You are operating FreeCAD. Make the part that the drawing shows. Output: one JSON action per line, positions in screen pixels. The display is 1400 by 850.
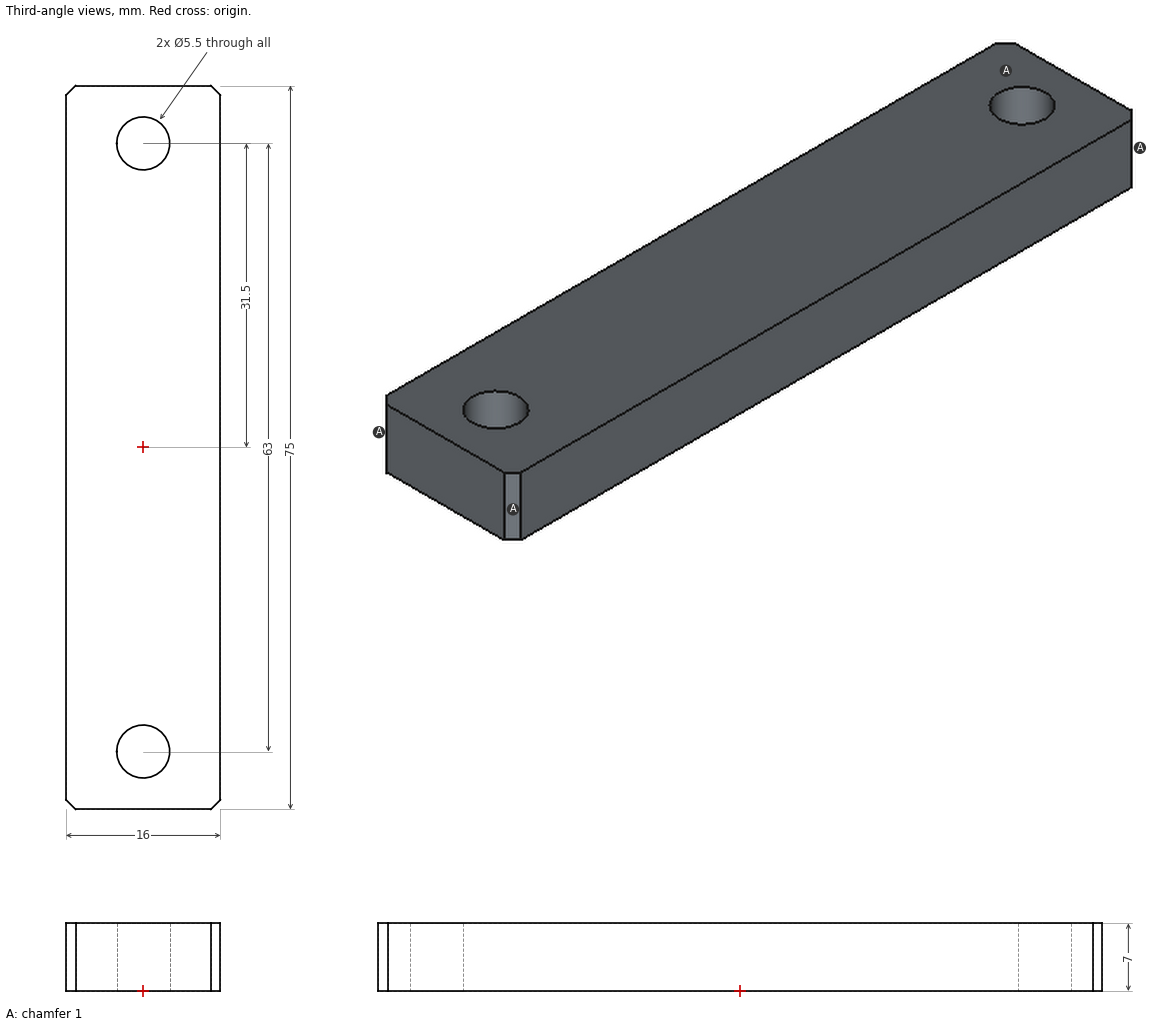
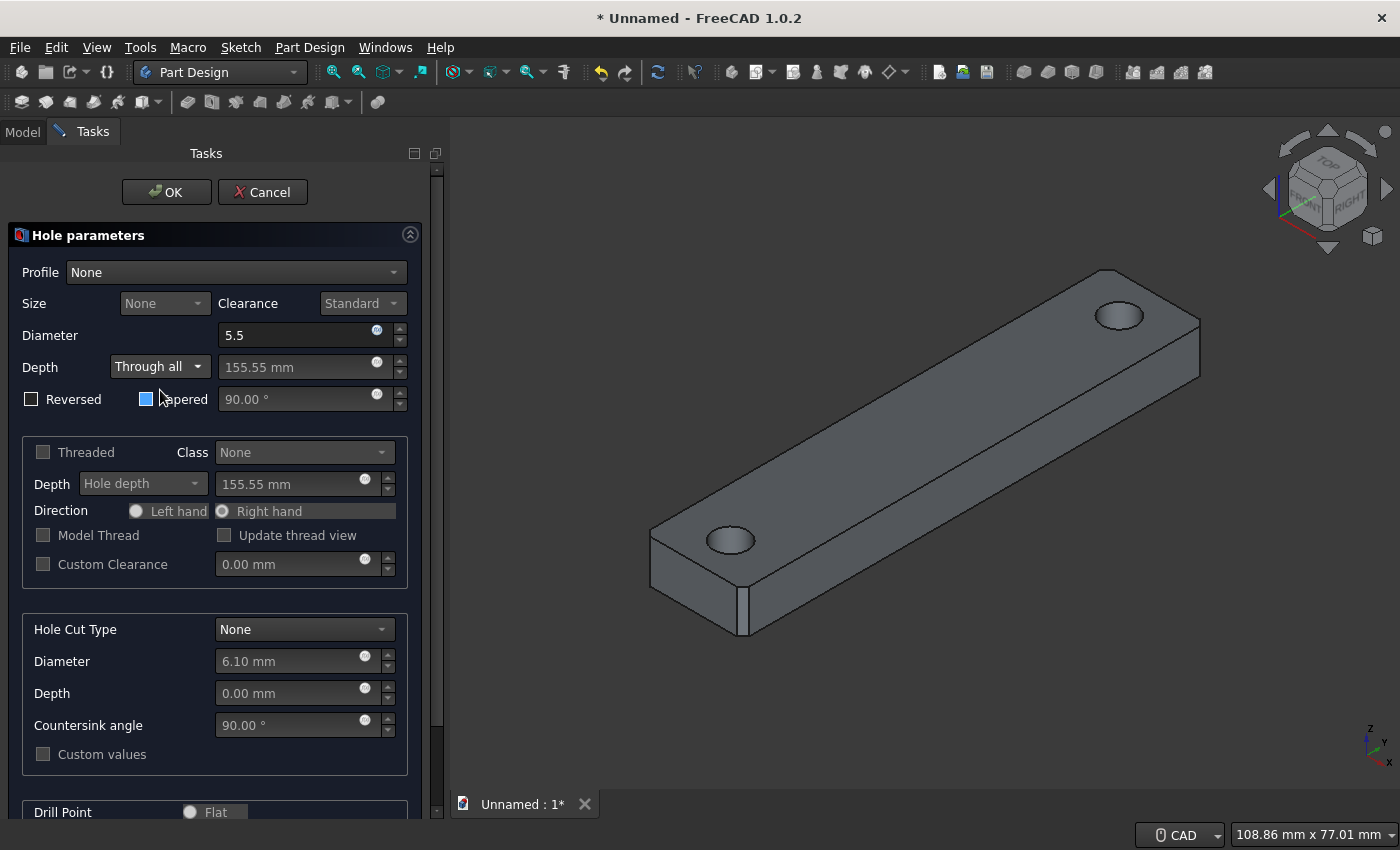
{"action": "left_click", "coordinate": [167, 192]}